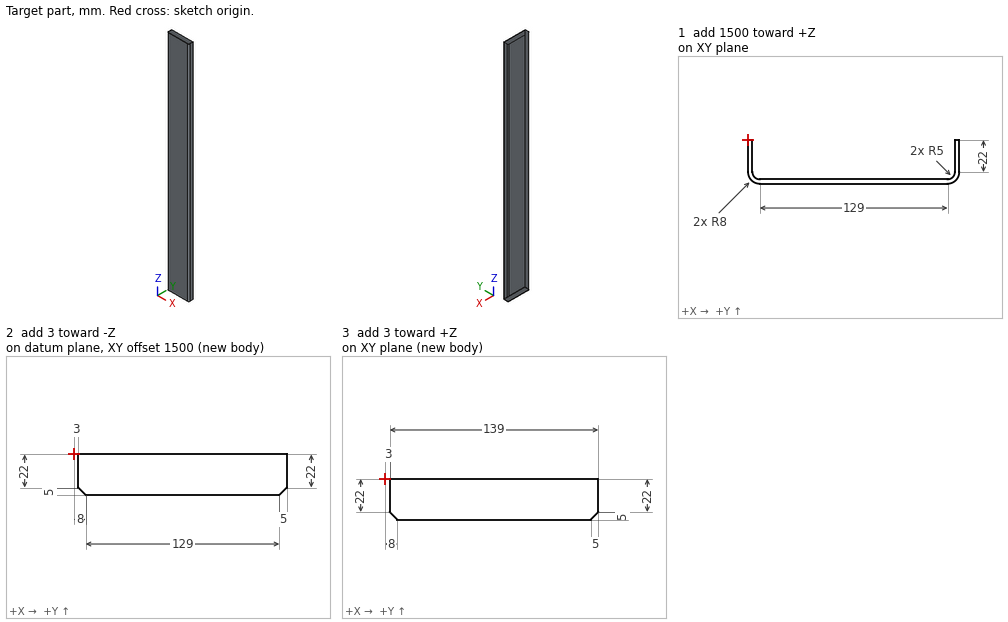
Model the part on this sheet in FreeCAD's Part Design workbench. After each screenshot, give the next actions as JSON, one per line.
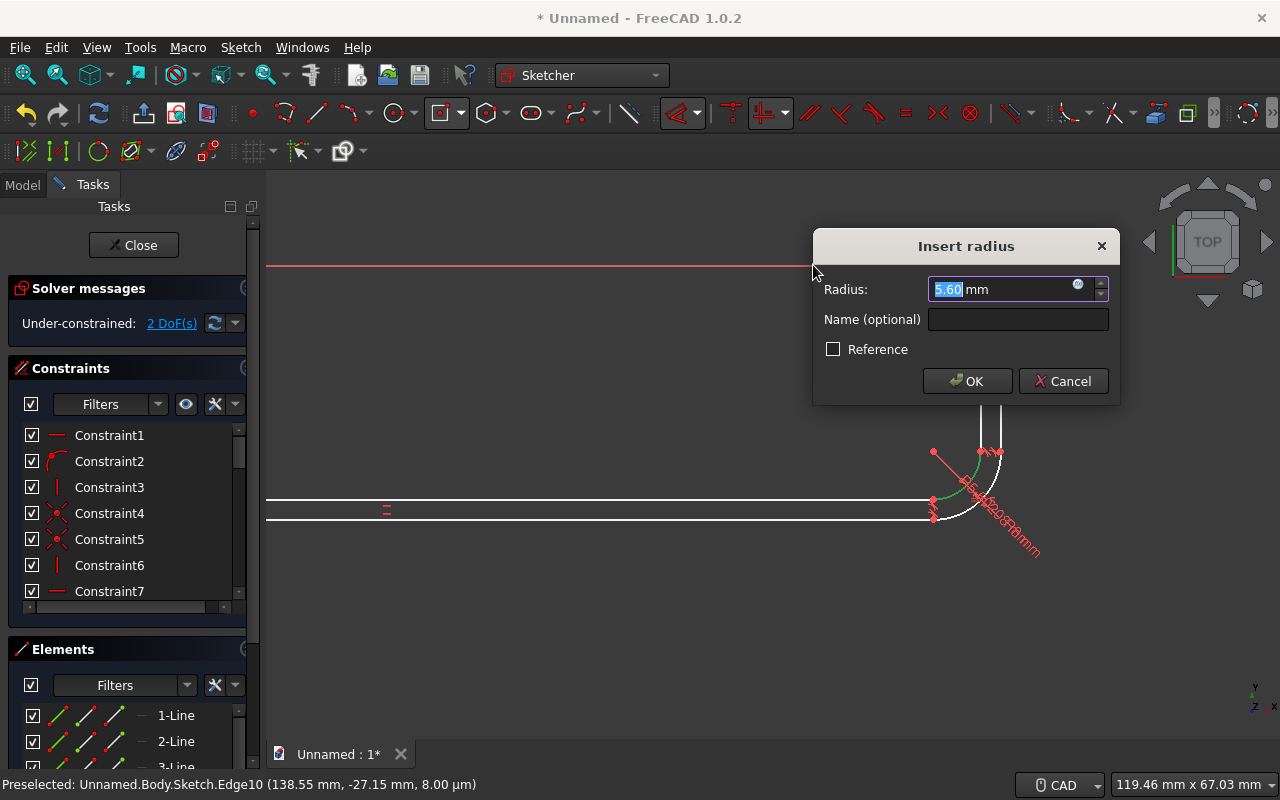
{"action": "type", "text": "5"}
{"action": "key", "text": "Return"}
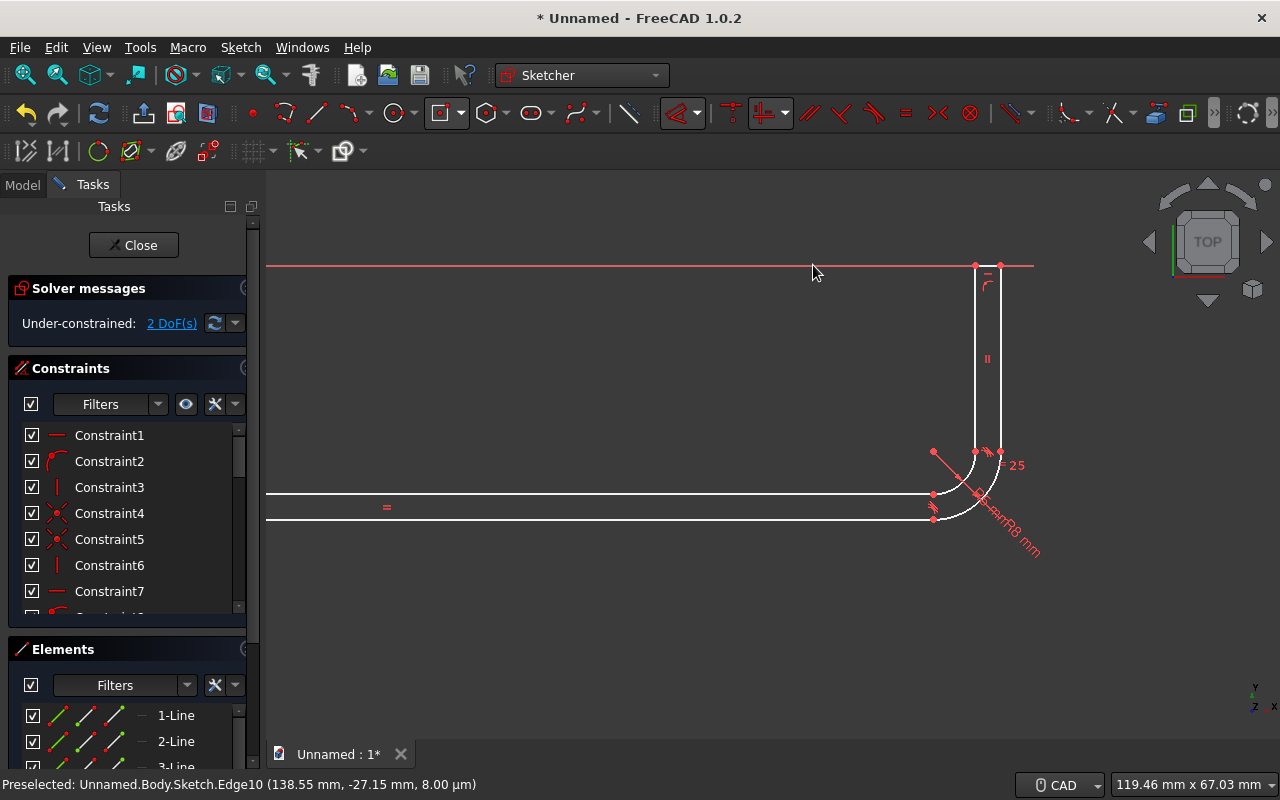
{"action": "left_click", "coordinate": [1001, 396]}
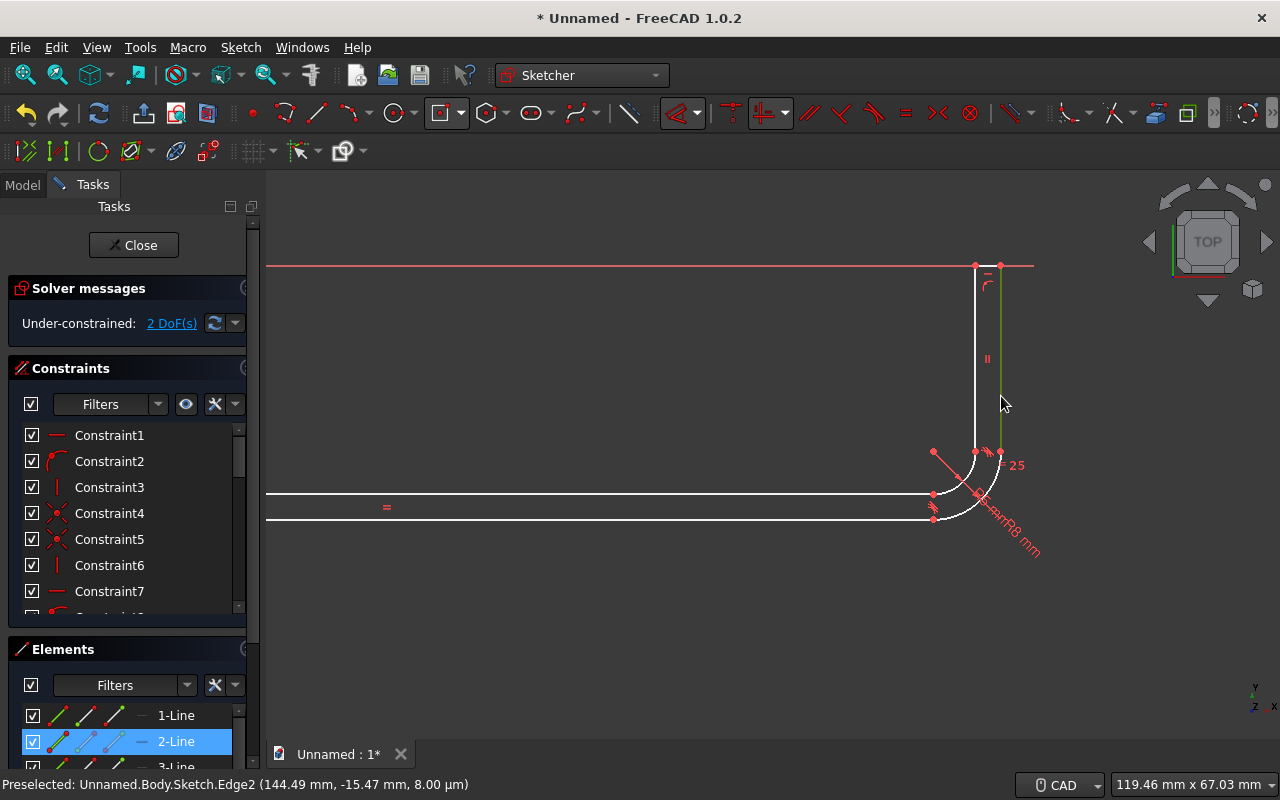
{"action": "key", "text": "i"}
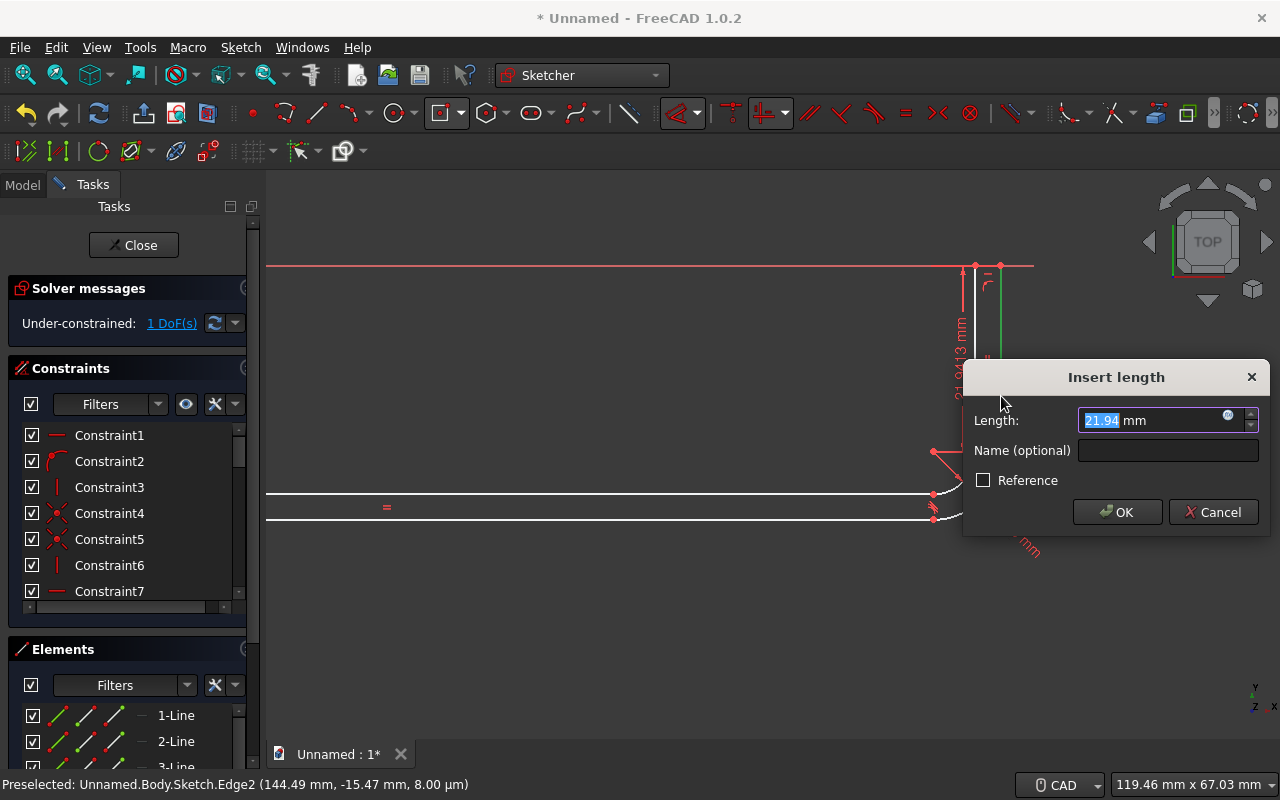
{"action": "type", "text": "22"}
{"action": "key", "text": "Return"}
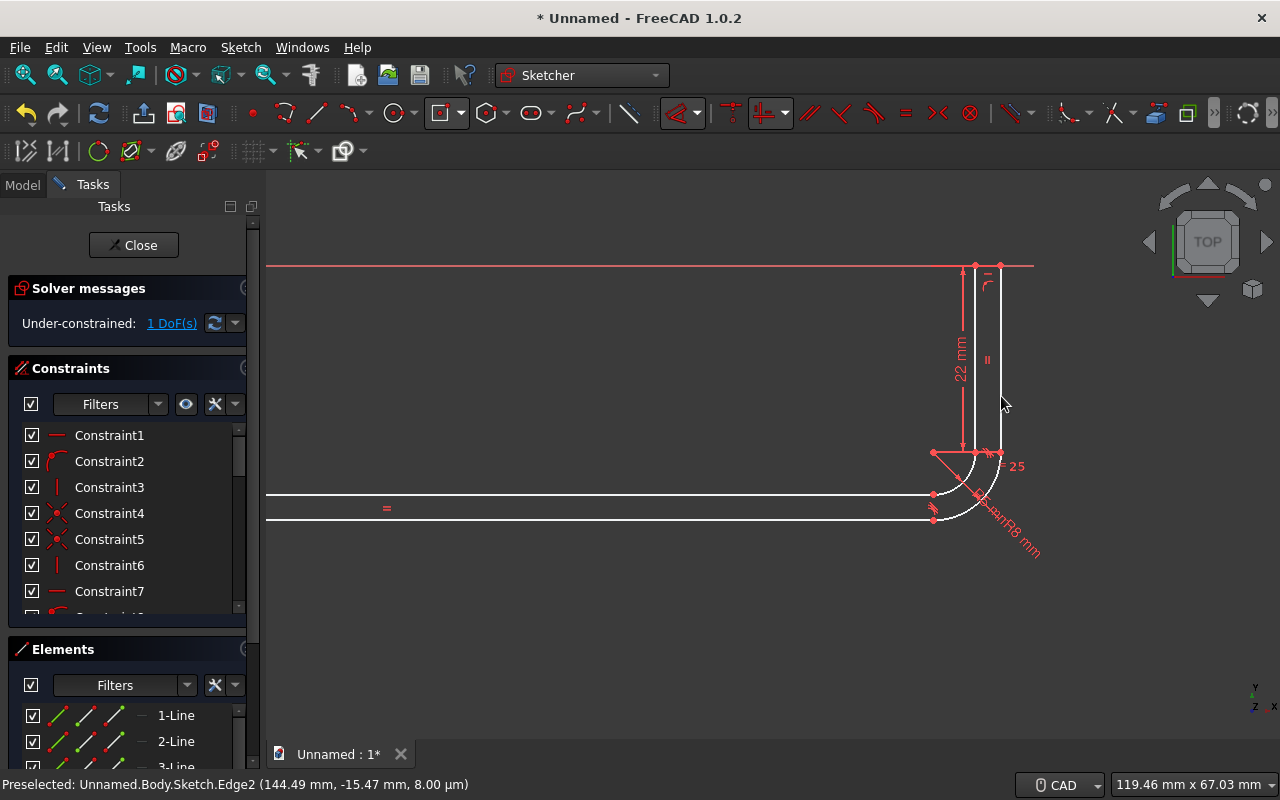
{"action": "left_click", "coordinate": [606, 520]}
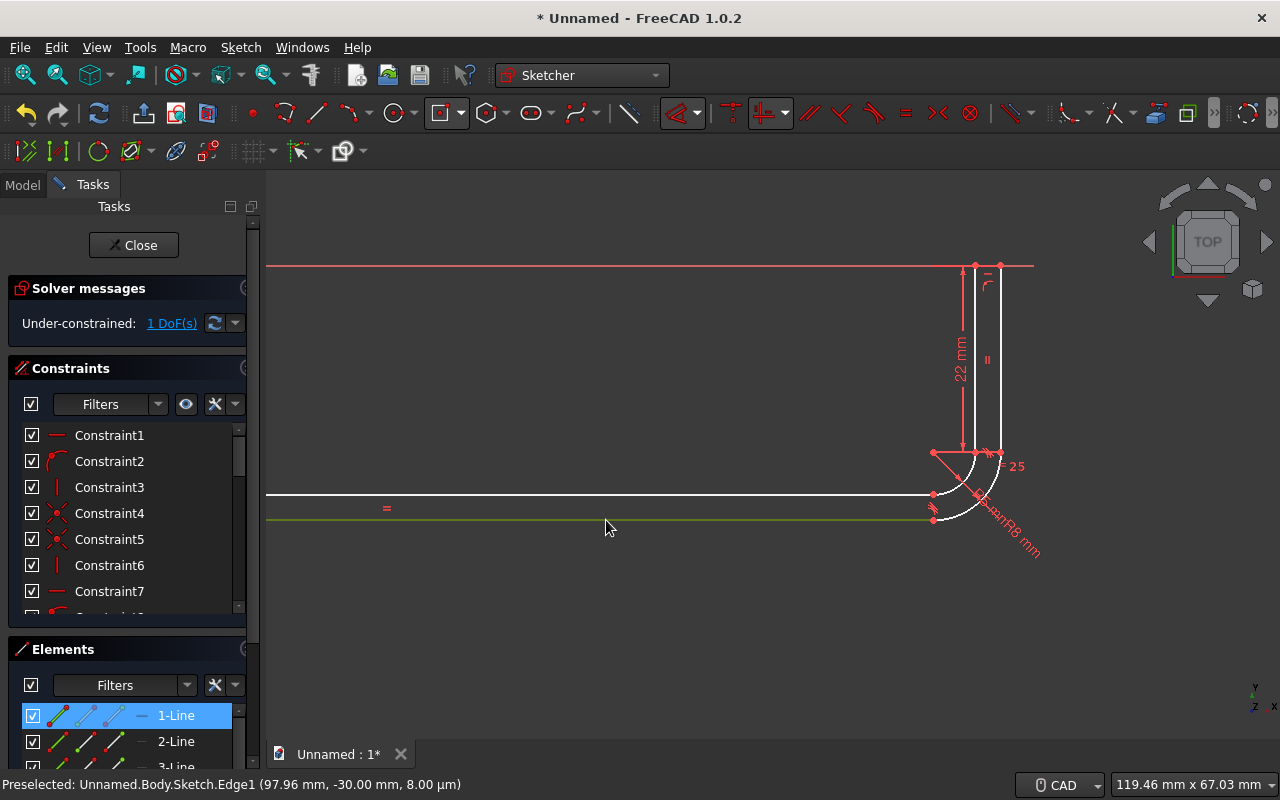
{"action": "key", "text": "l"}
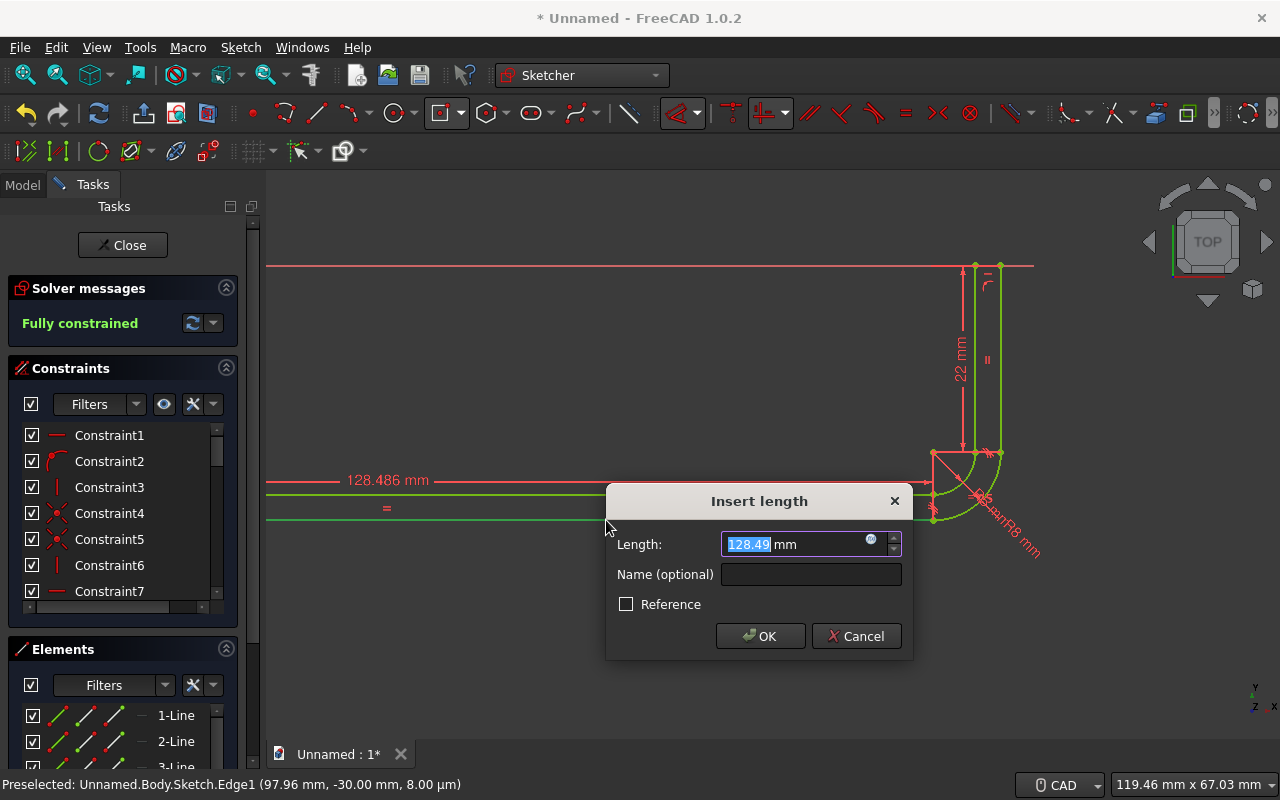
{"action": "type", "text": "129"}
{"action": "key", "text": "Return"}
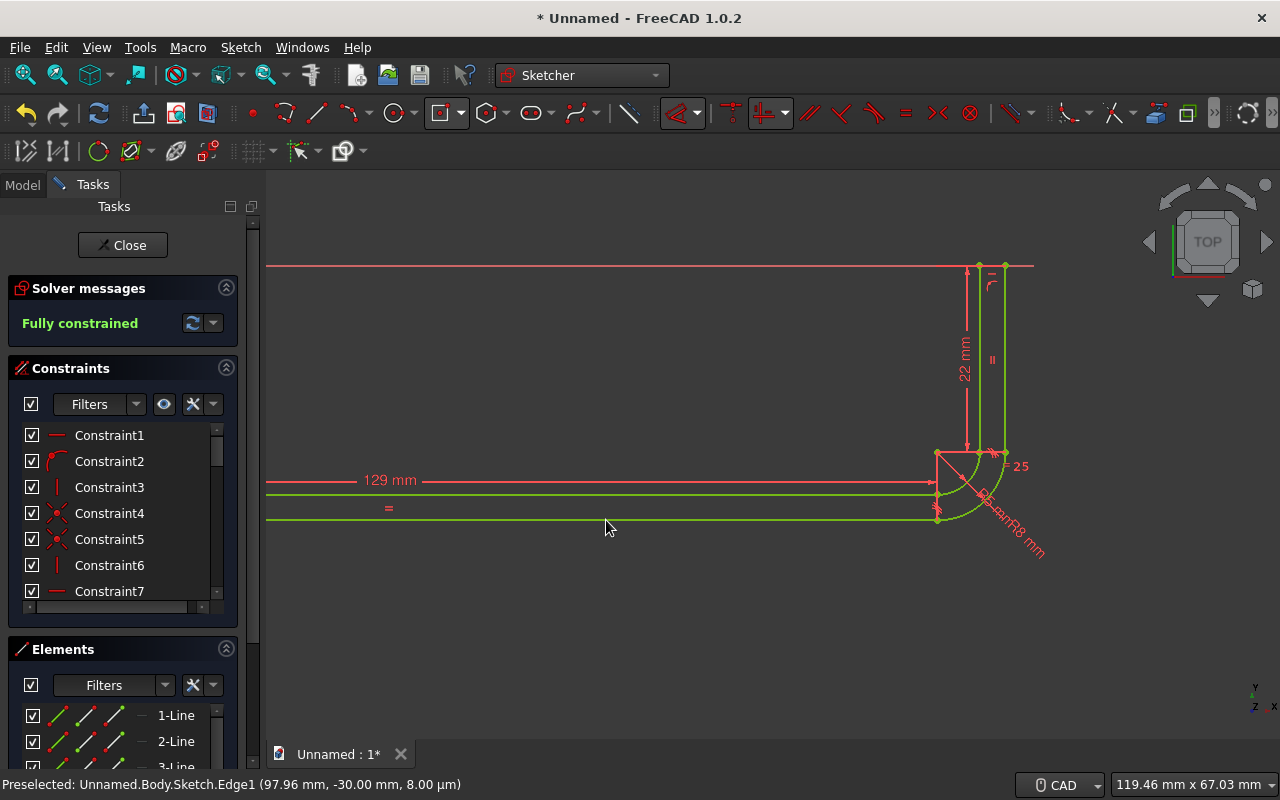
{"action": "left_click", "coordinate": [123, 245]}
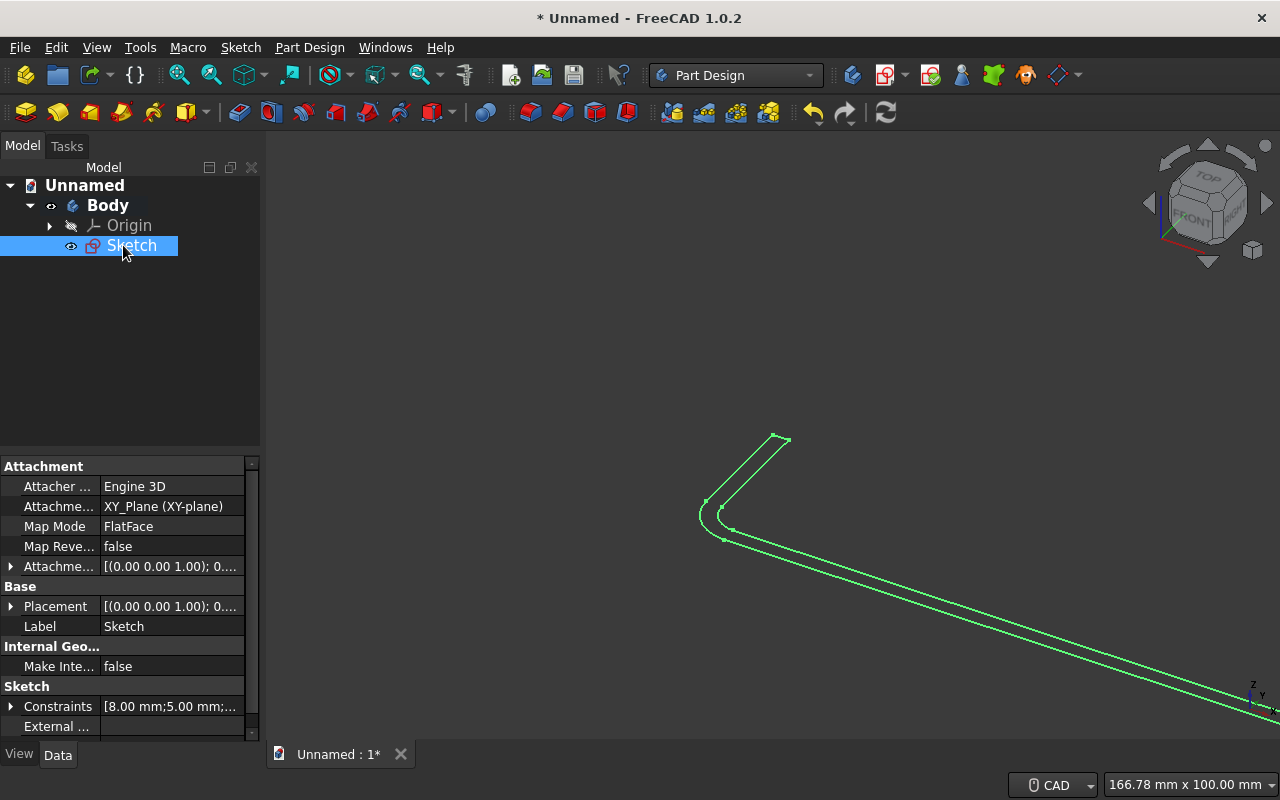
{"action": "left_click", "coordinate": [26, 112]}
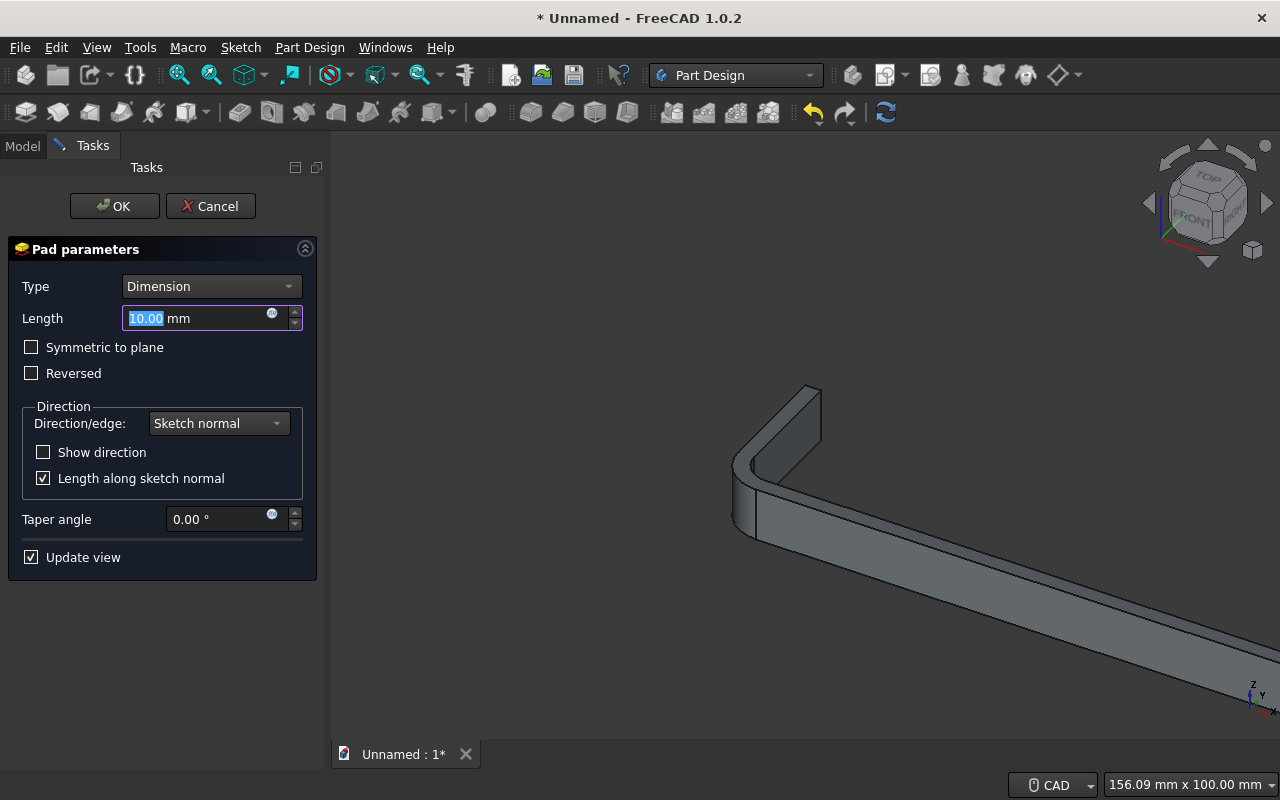
{"action": "type", "text": "1500"}
{"action": "key", "text": "Tab"}